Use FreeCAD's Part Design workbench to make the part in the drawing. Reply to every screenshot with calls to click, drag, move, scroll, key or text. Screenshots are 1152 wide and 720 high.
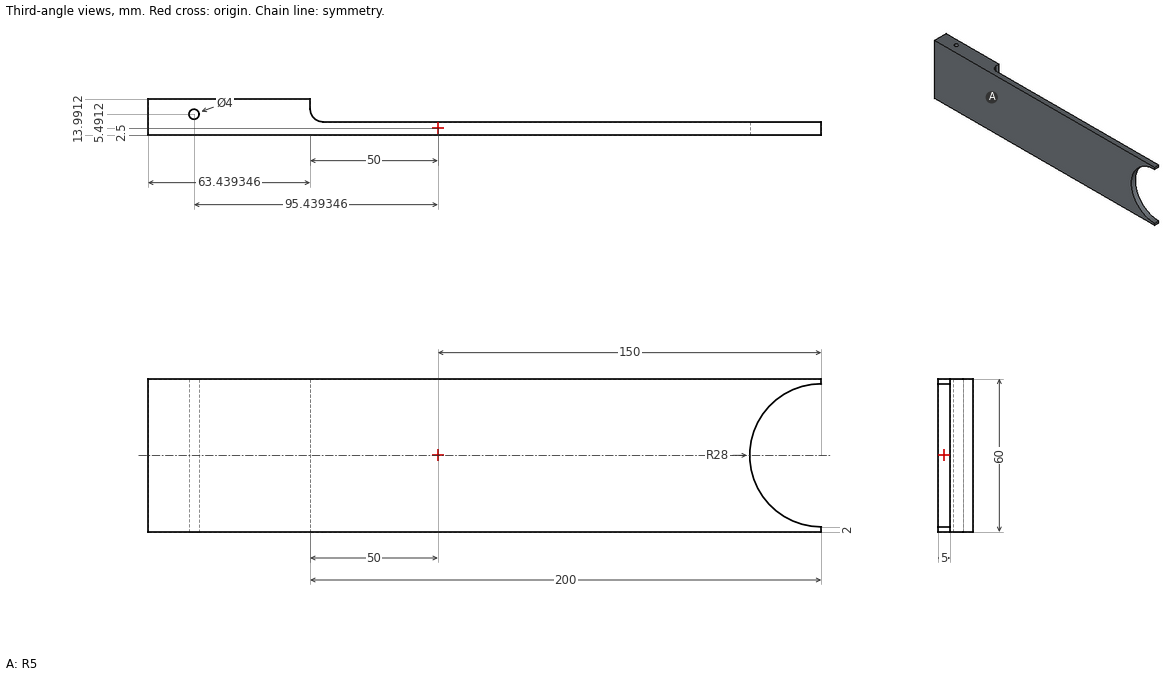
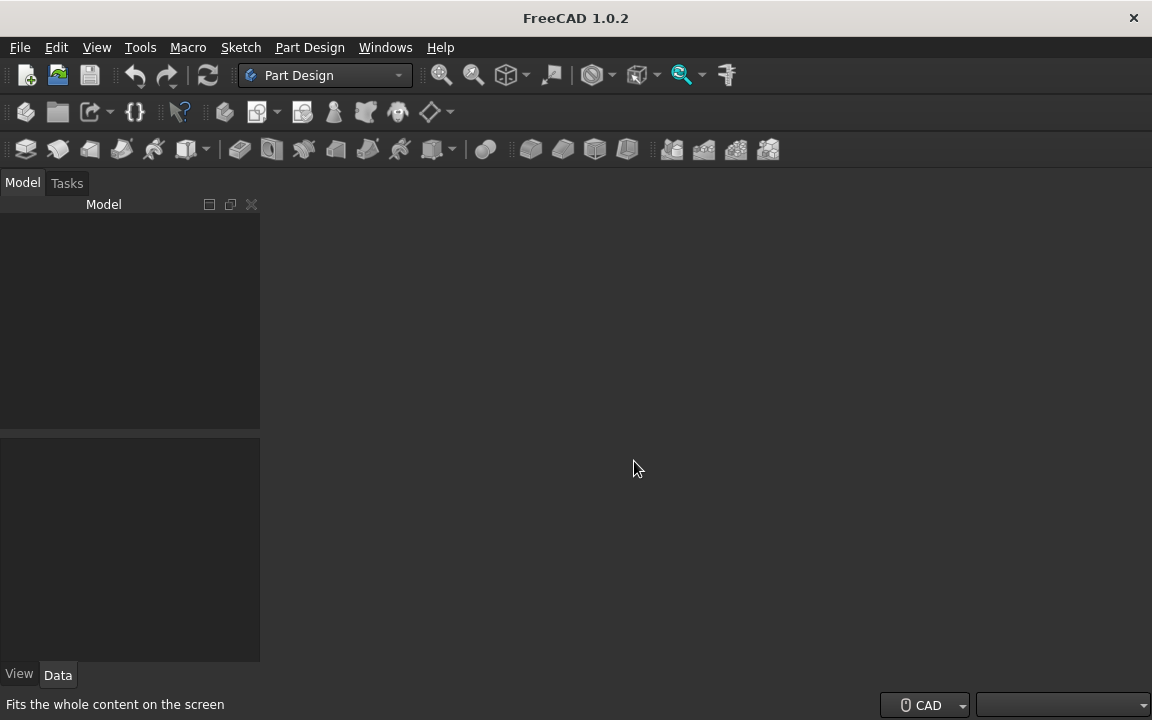
click(26, 76)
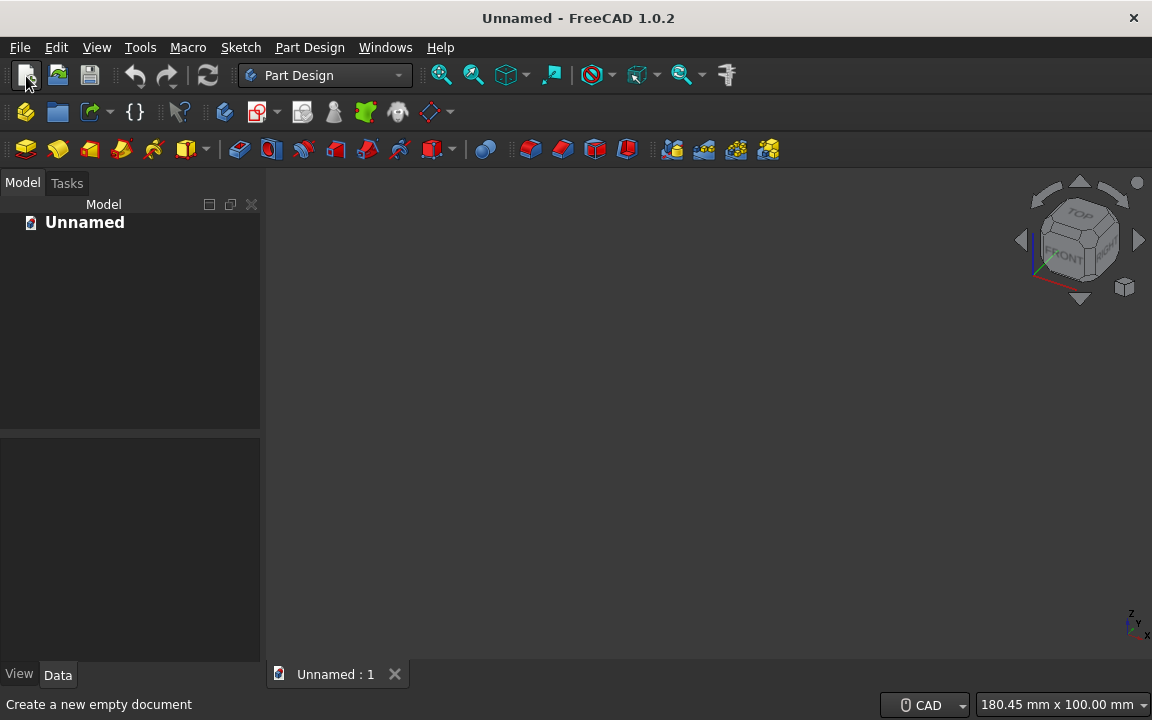
click(258, 112)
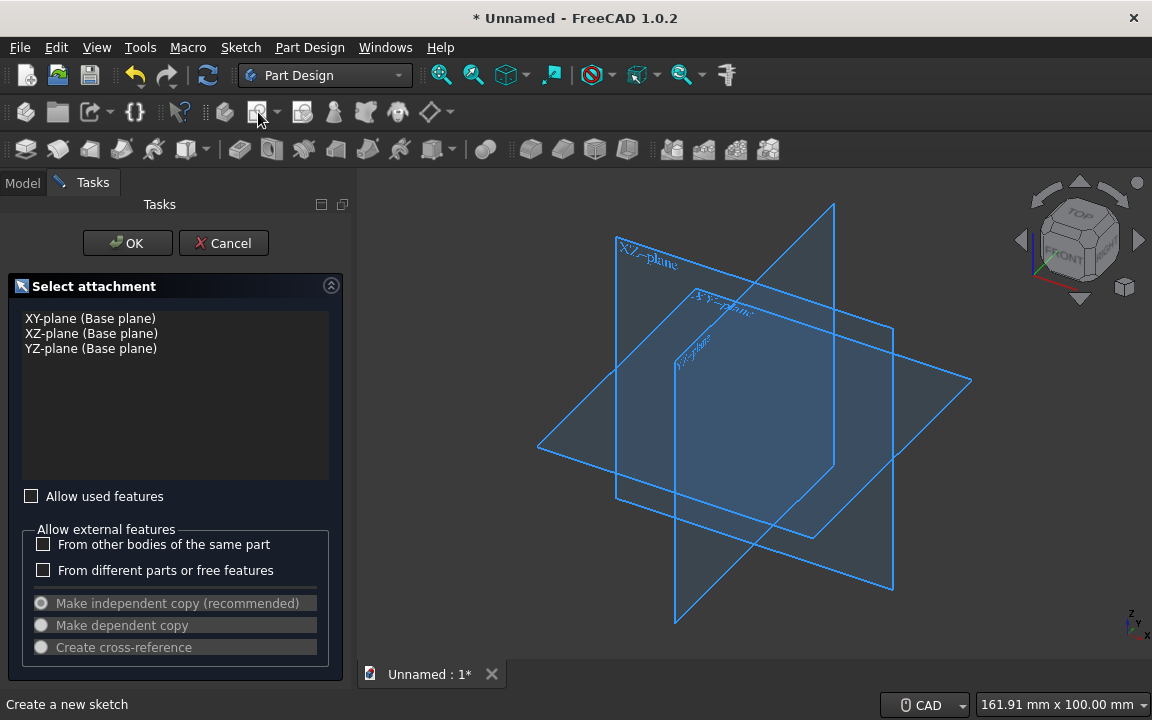
click(82, 334)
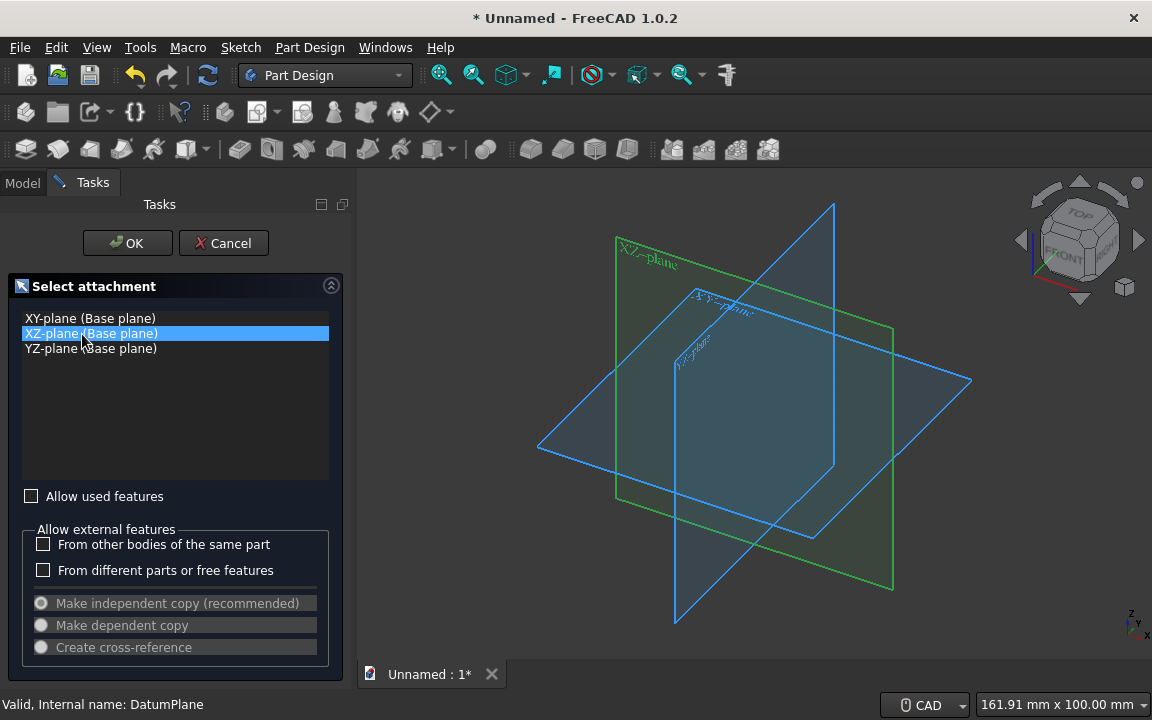
click(128, 243)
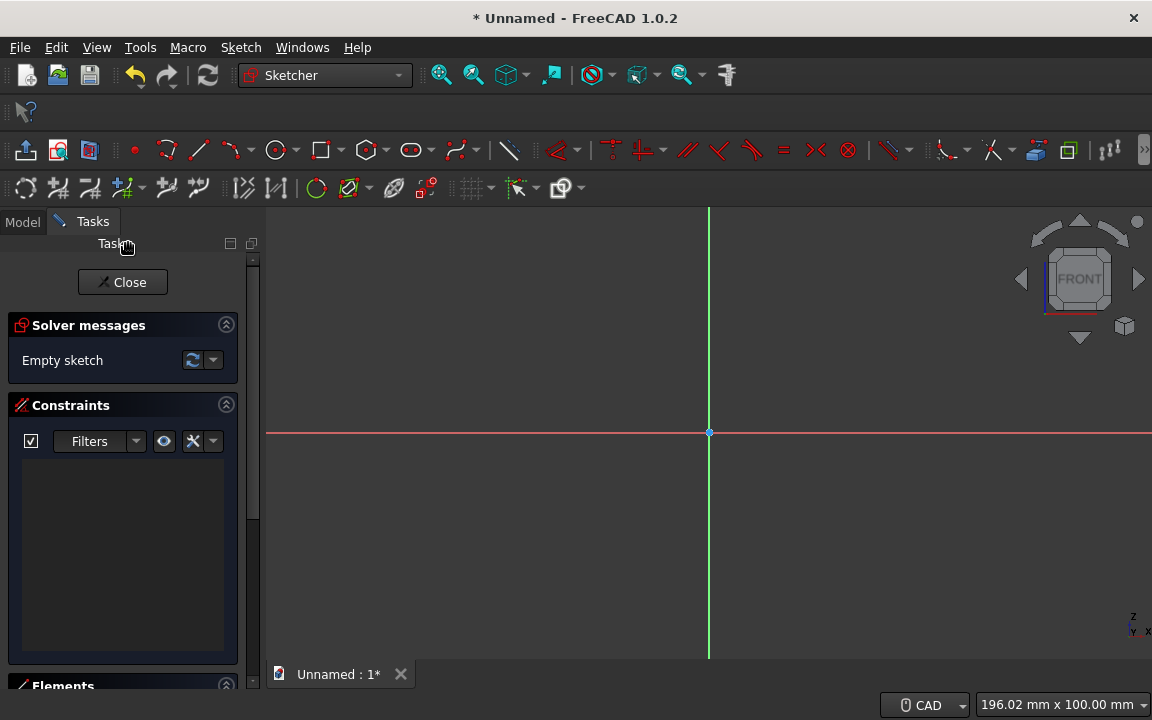
scroll(294, 433, down, 3)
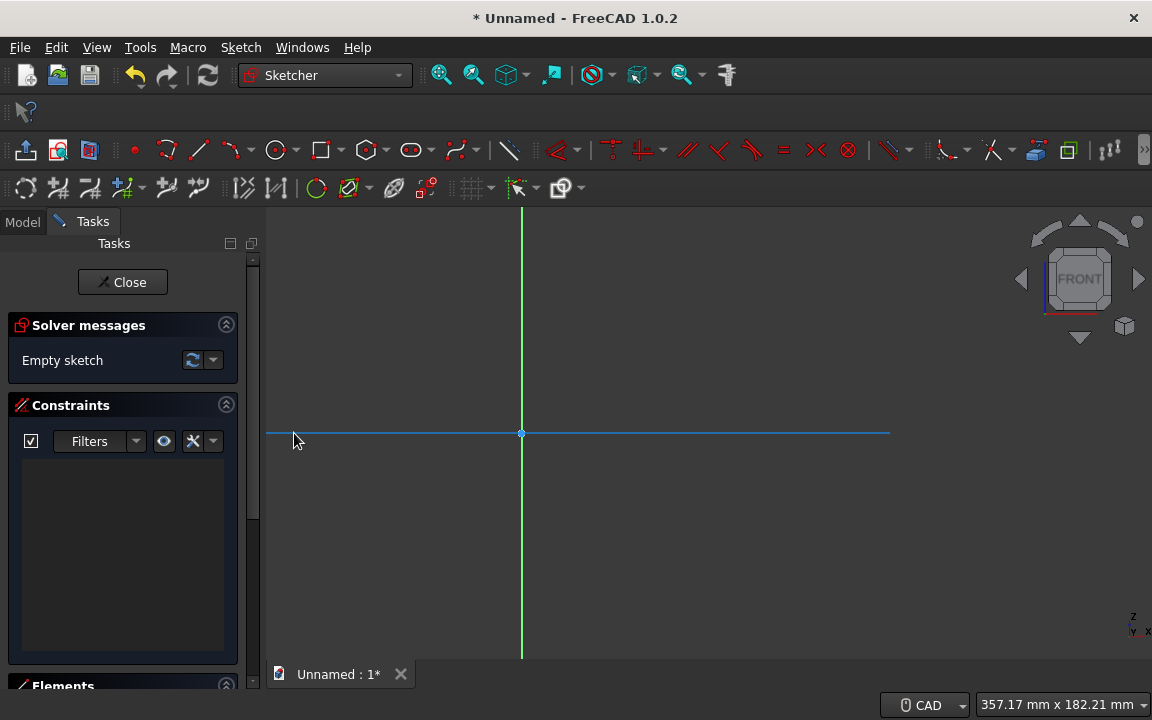
key(g)
key(m)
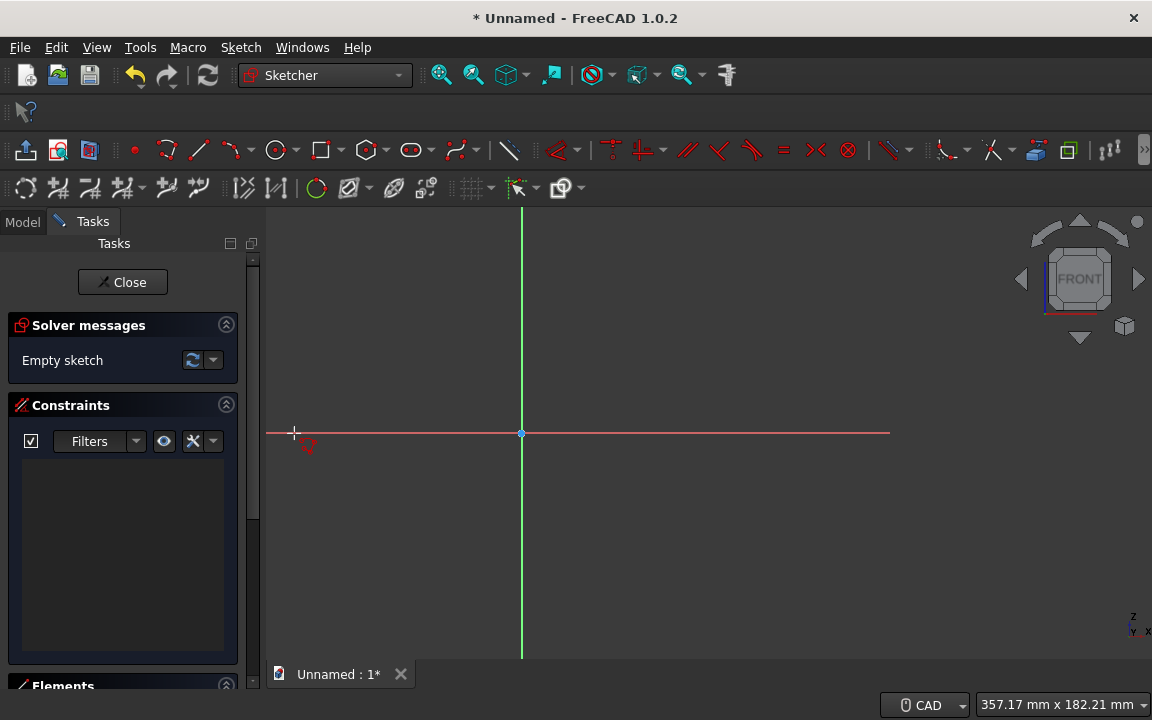
click(894, 503)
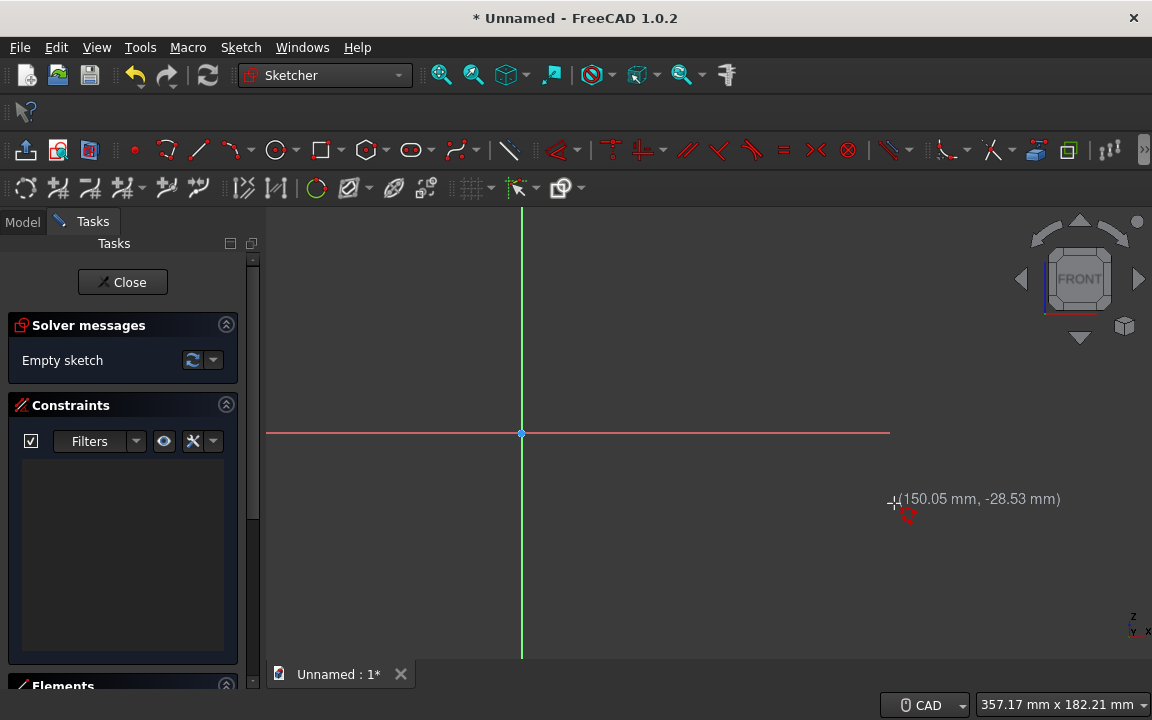
scroll(894, 508, up, 6)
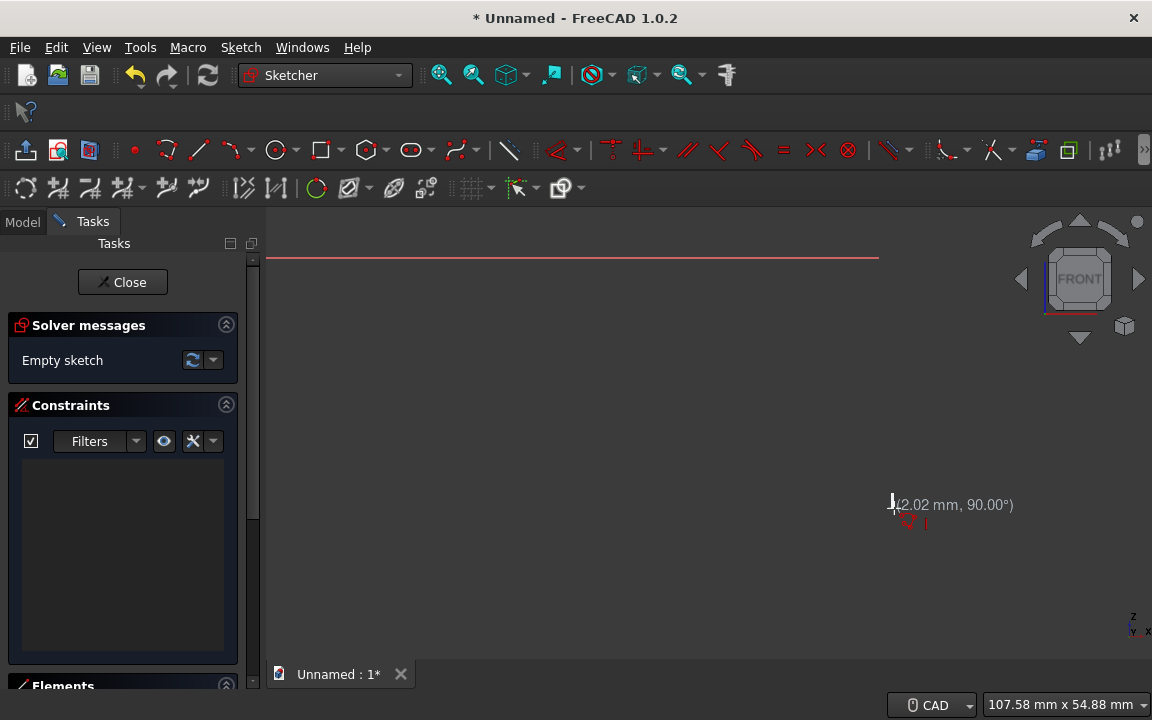
click(892, 505)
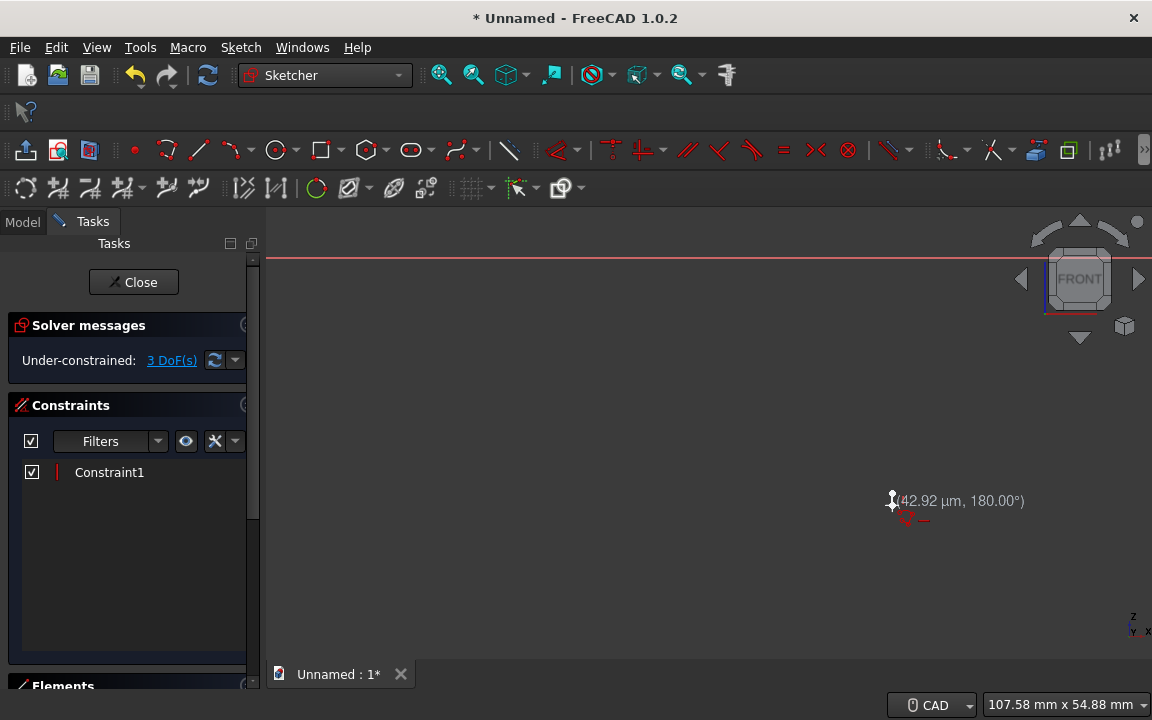
scroll(887, 508, down, 6)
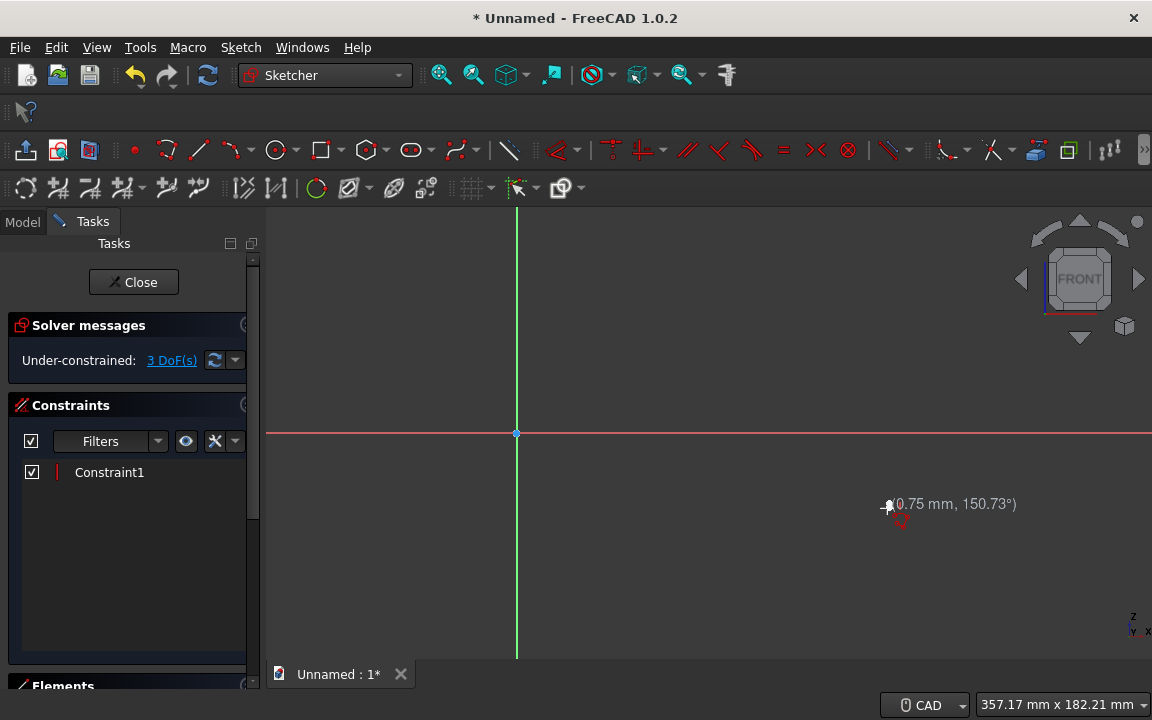
click(393, 508)
click(393, 359)
click(889, 359)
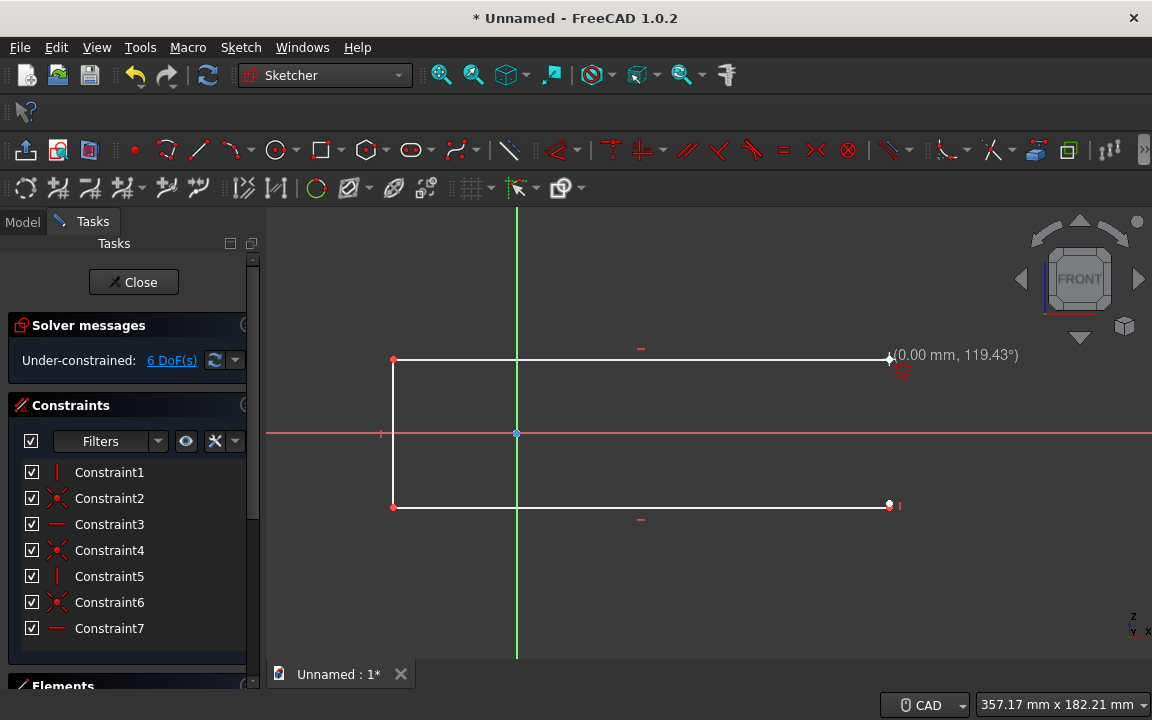
scroll(889, 364, up, 6)